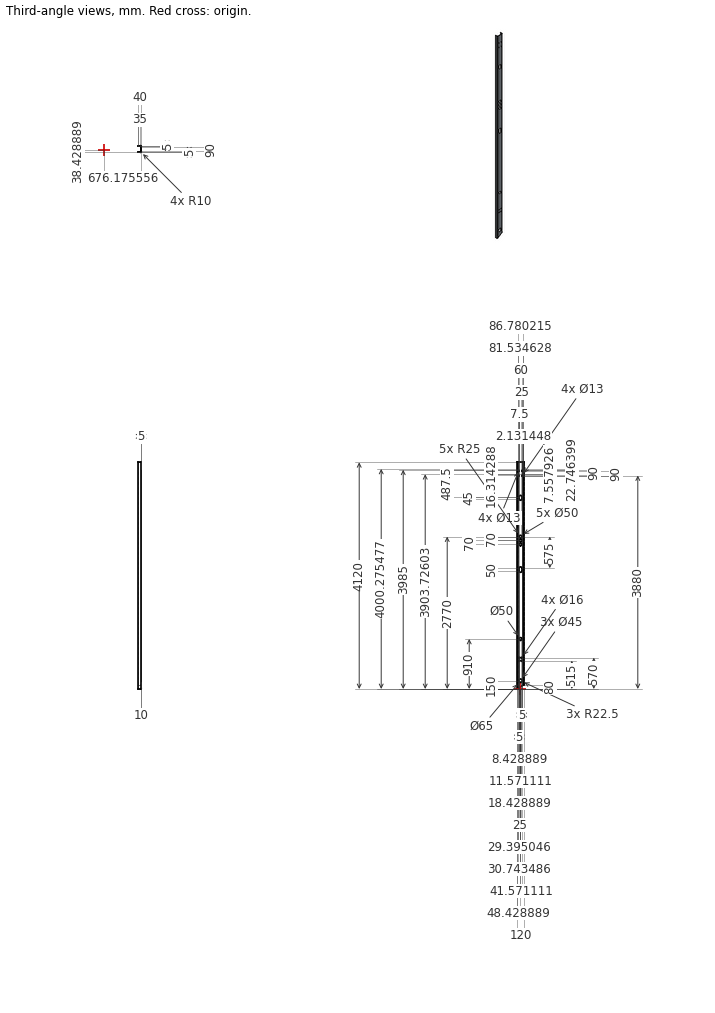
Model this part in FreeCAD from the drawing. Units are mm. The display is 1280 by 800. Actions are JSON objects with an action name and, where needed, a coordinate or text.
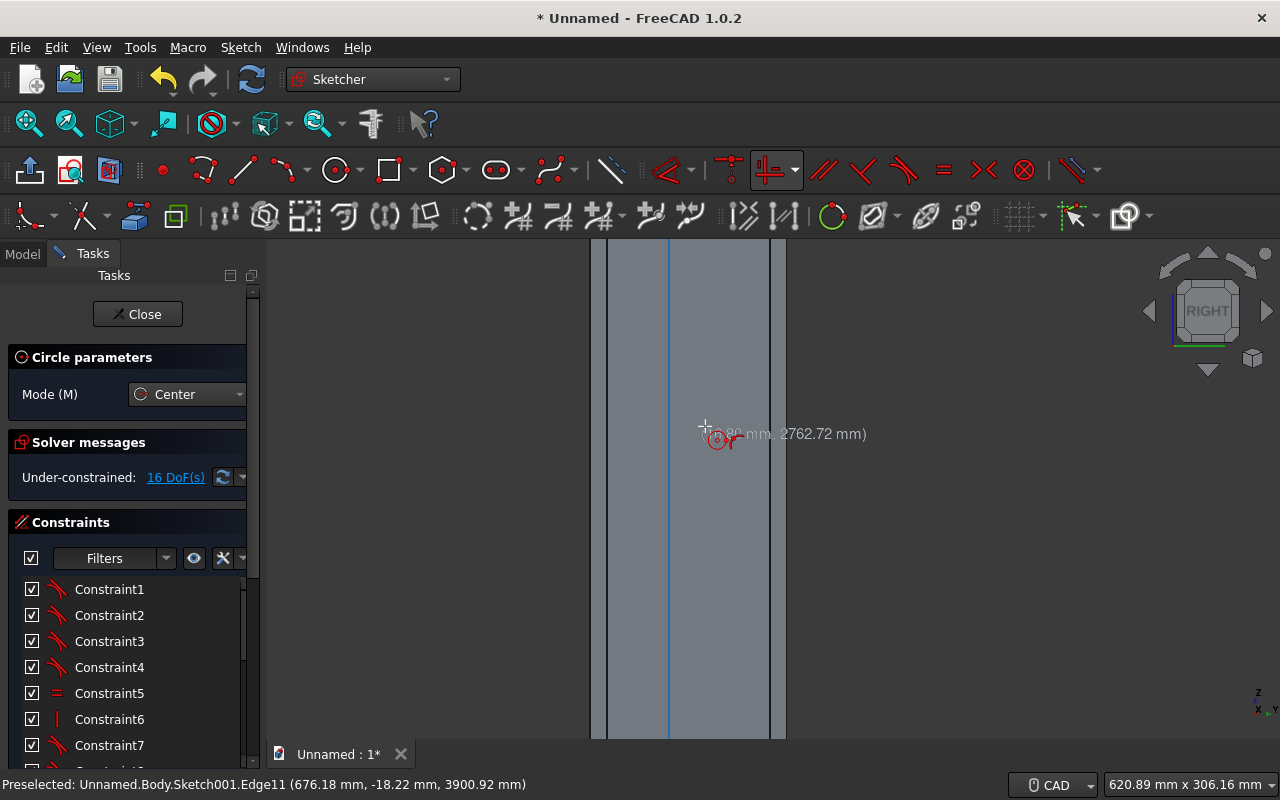
{"action": "left_click", "coordinate": [688, 427]}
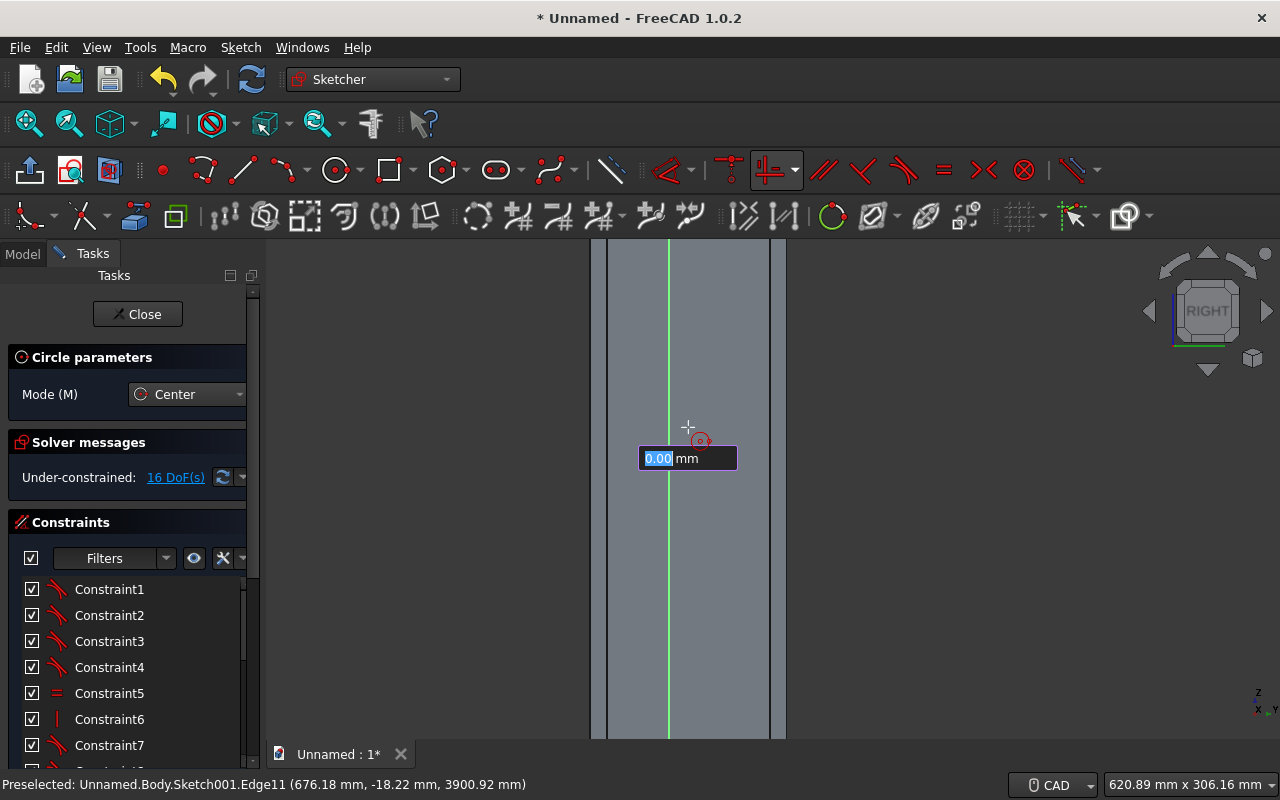
{"action": "scroll", "coordinate": [705, 426], "scroll_direction": "down", "scroll_amount": 15}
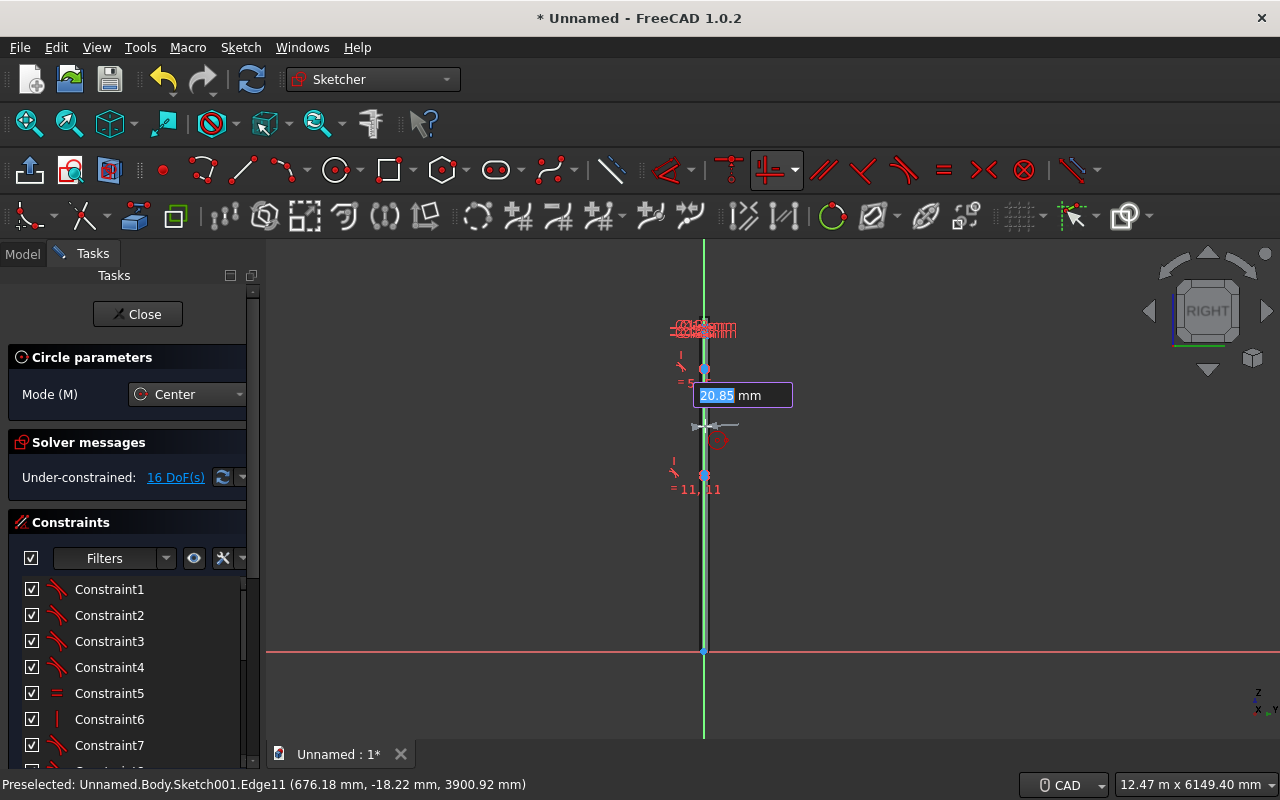
{"action": "scroll", "coordinate": [706, 425], "scroll_direction": "up", "scroll_amount": 10}
{"action": "mouse_move", "coordinate": [703, 422]}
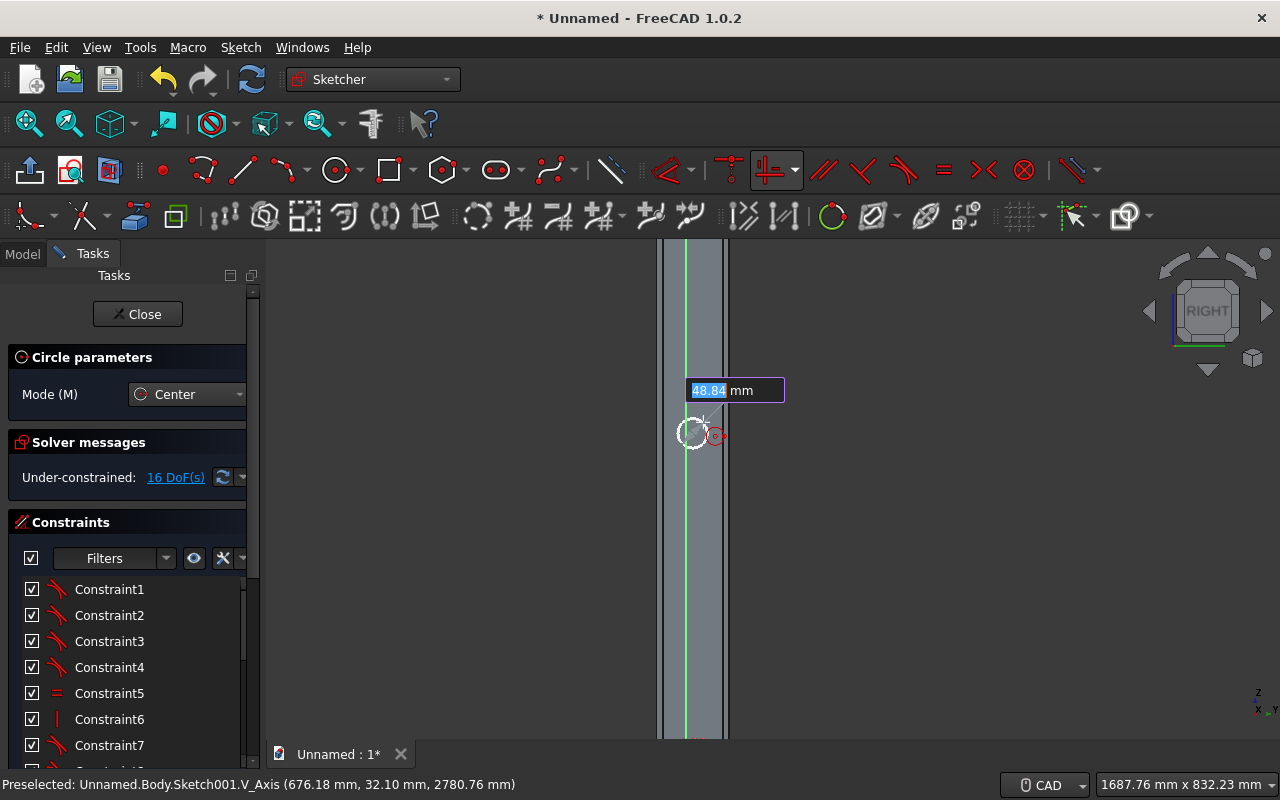
{"action": "type", "text": "50"}
{"action": "key", "text": "Return"}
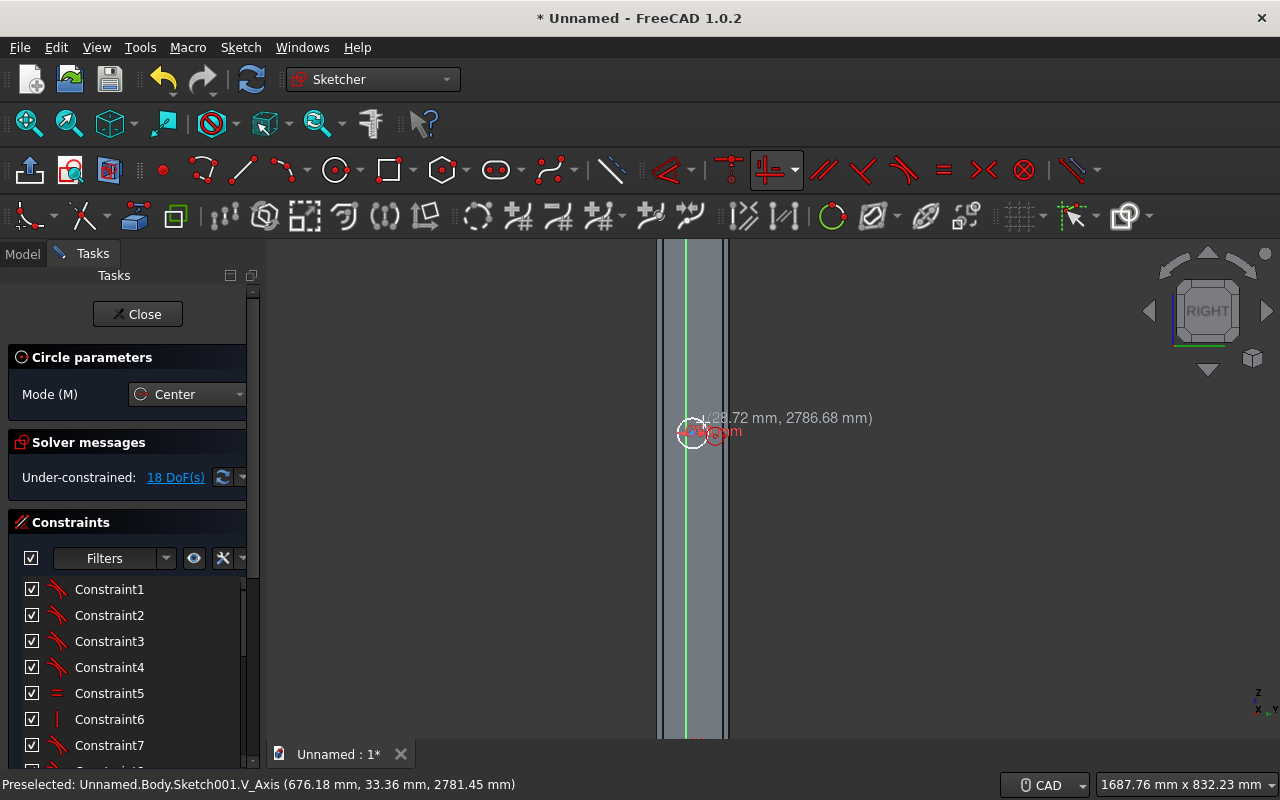
{"action": "scroll", "coordinate": [693, 475], "scroll_direction": "up", "scroll_amount": 5}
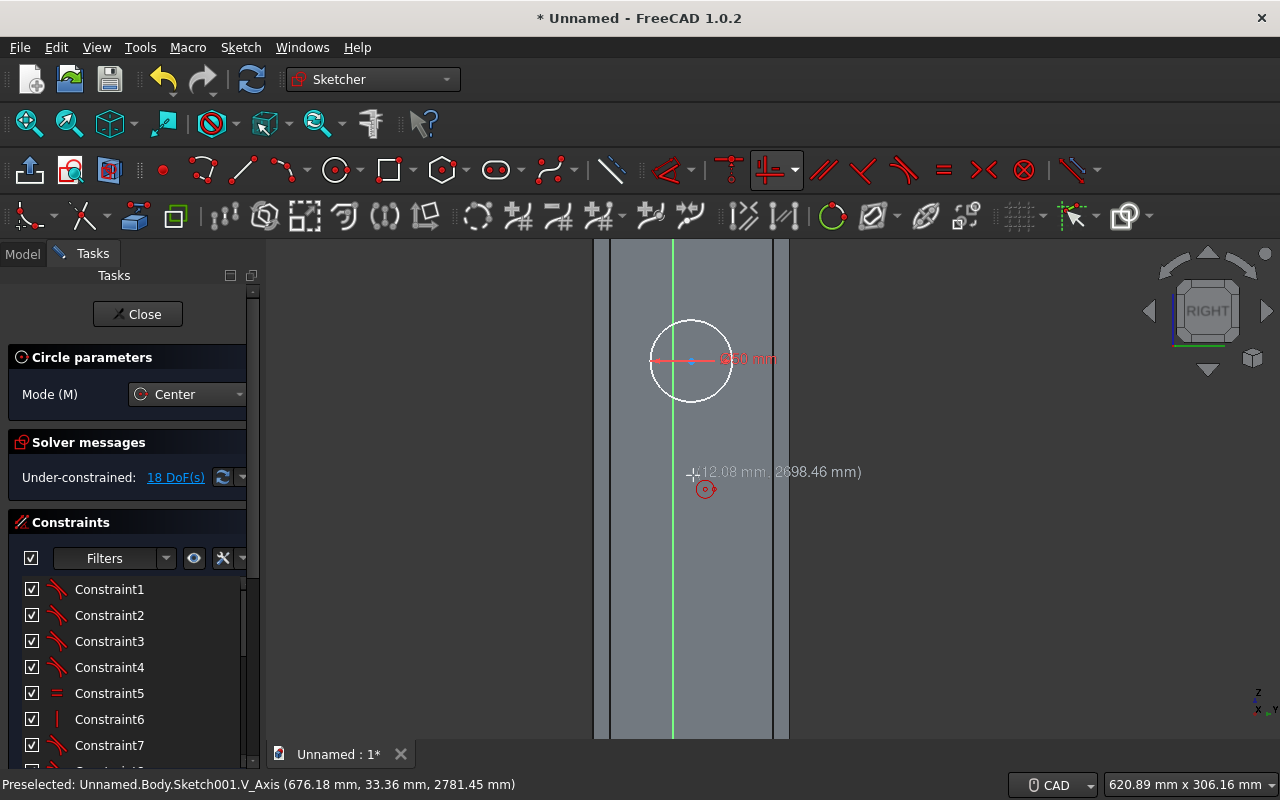
{"action": "left_click", "coordinate": [691, 474]}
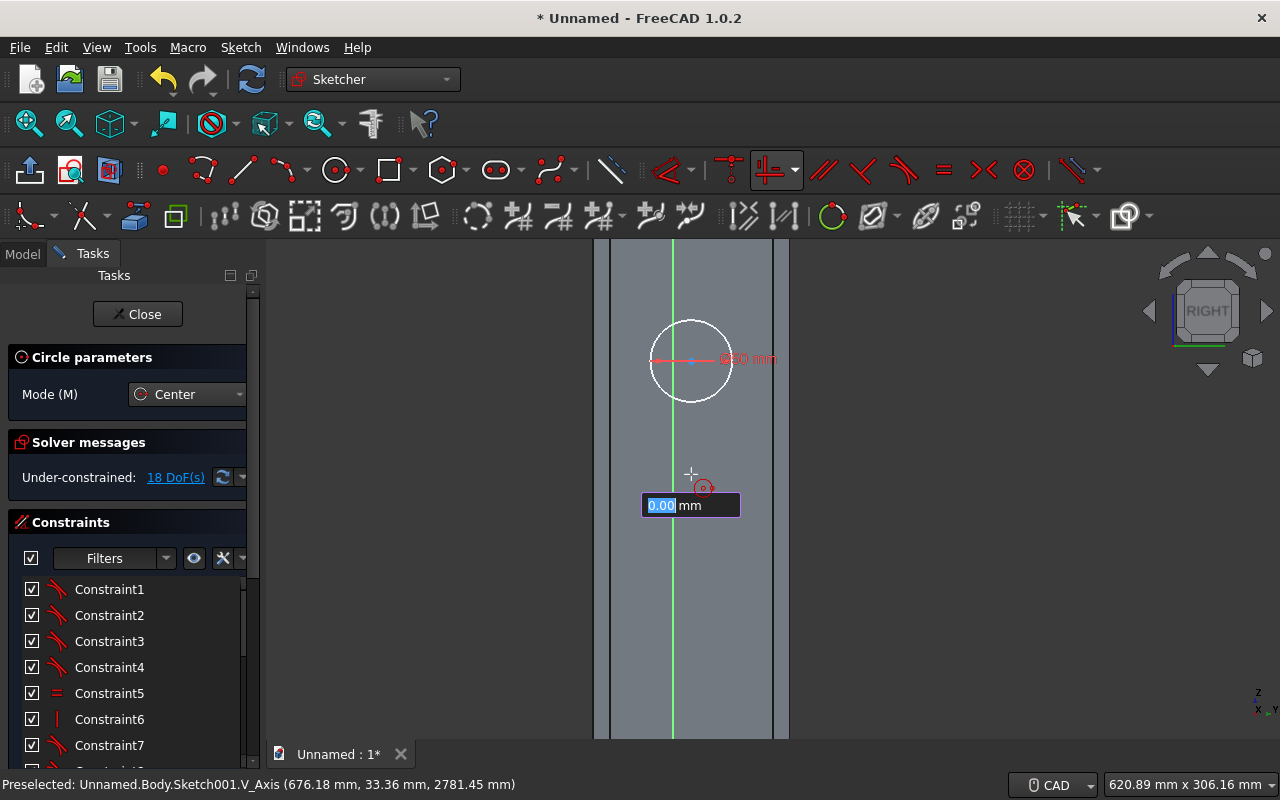
{"action": "scroll", "coordinate": [705, 430], "scroll_direction": "down", "scroll_amount": 15}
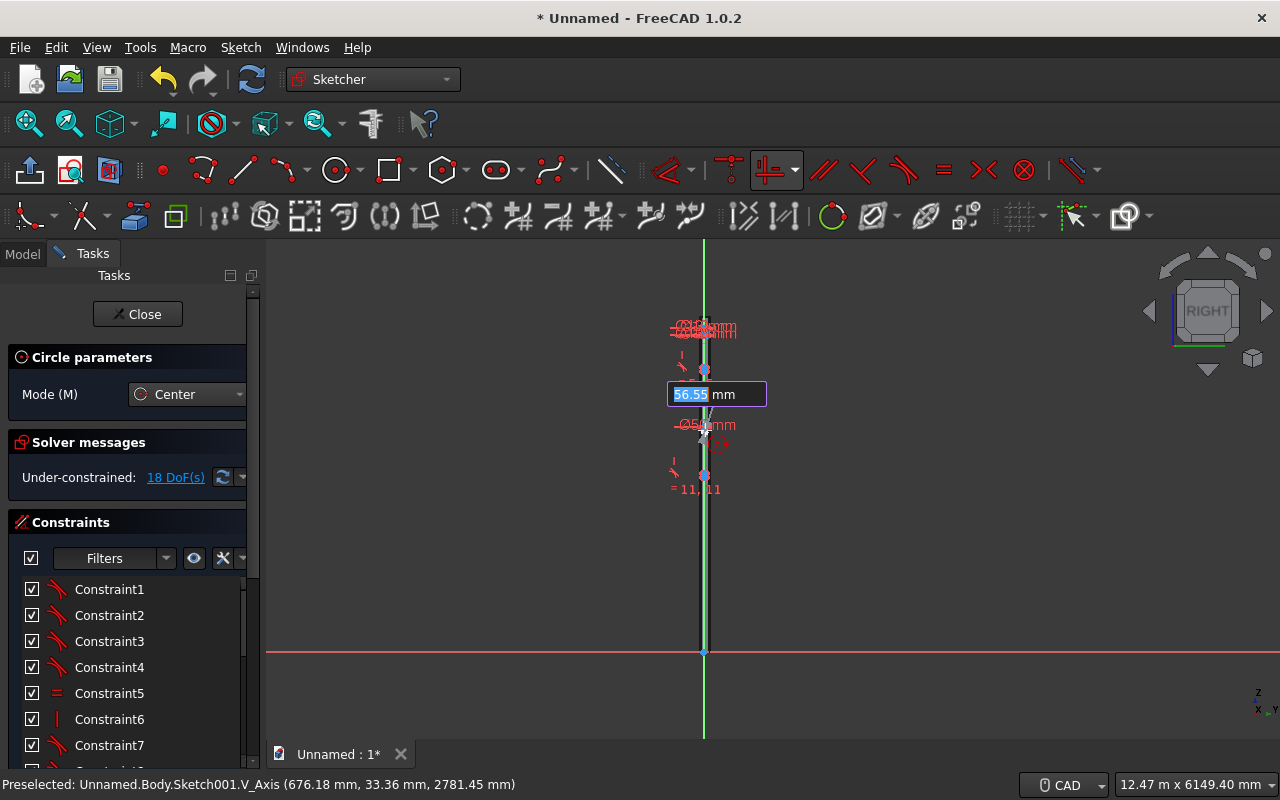
{"action": "scroll", "coordinate": [706, 431], "scroll_direction": "up", "scroll_amount": 10}
{"action": "mouse_move", "coordinate": [705, 430]}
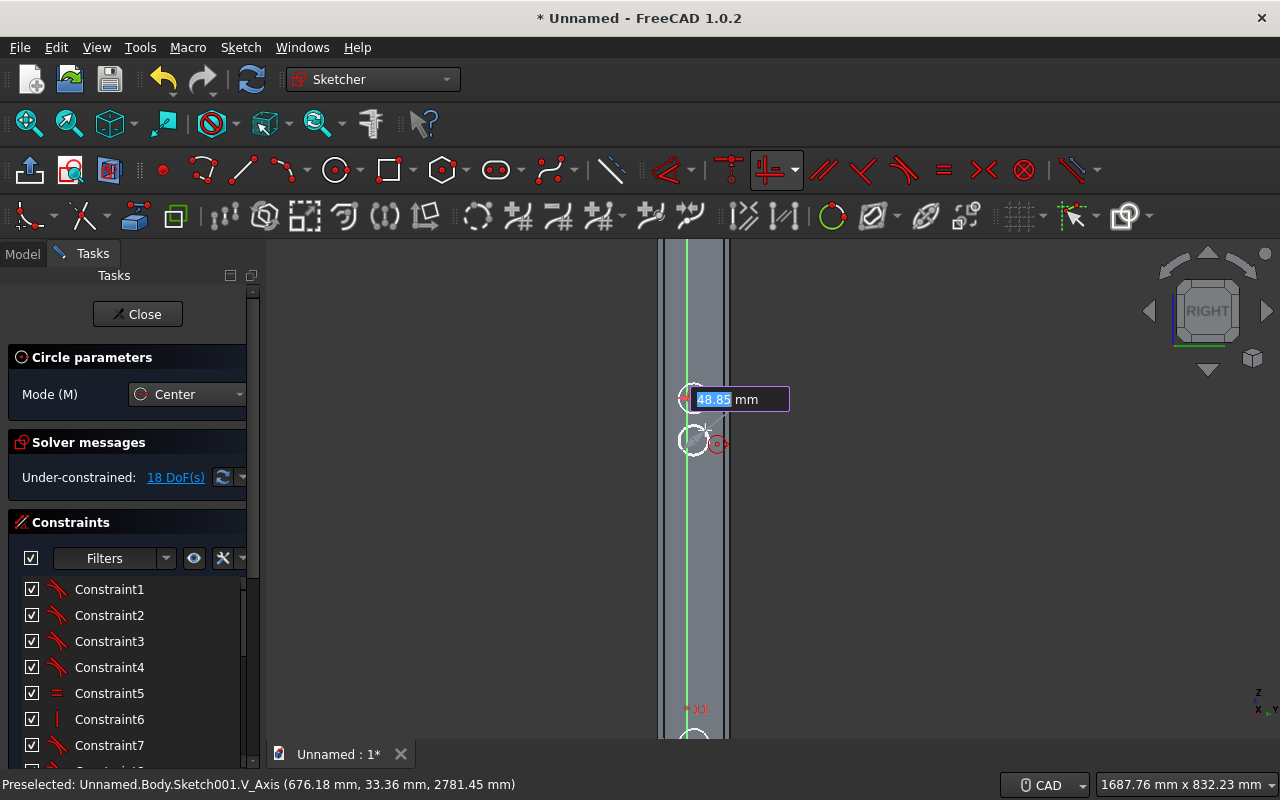
{"action": "type", "text": "50"}
{"action": "key", "text": "Return"}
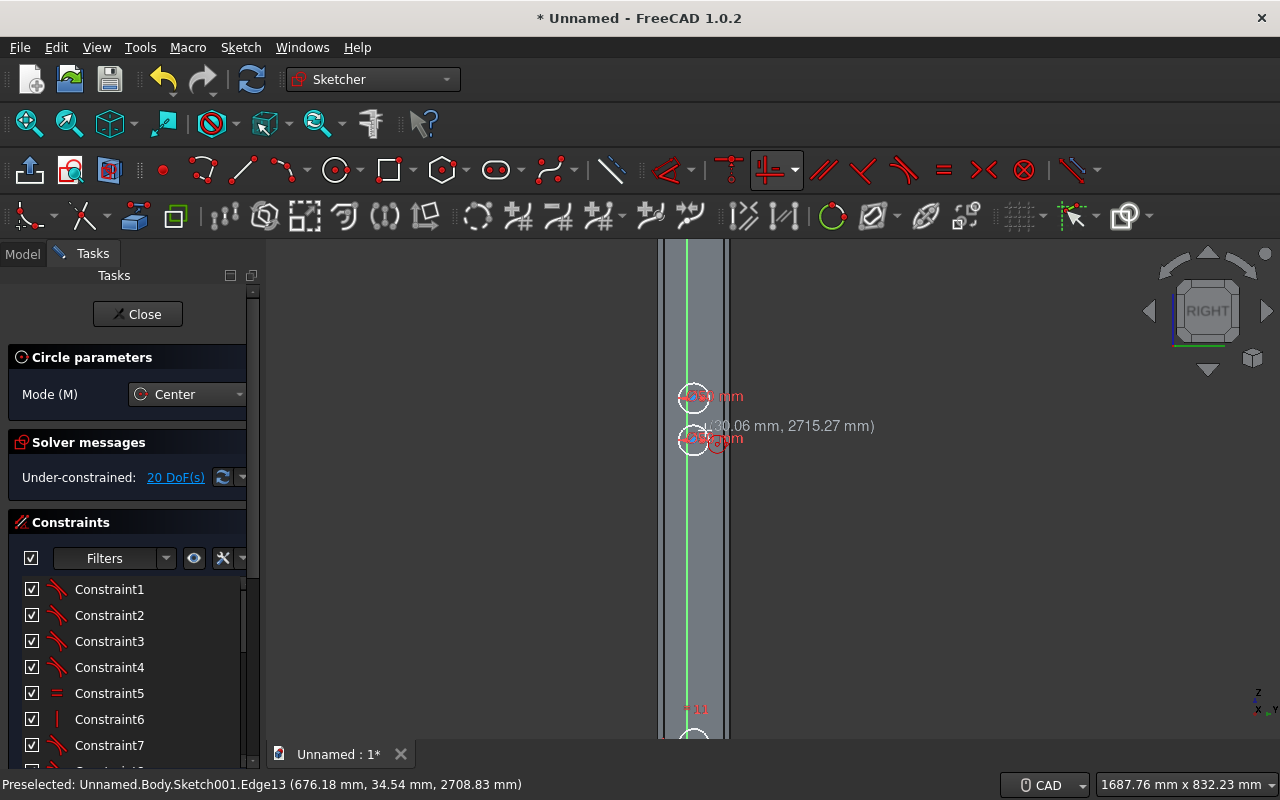
{"action": "scroll", "coordinate": [694, 482], "scroll_direction": "up", "scroll_amount": 5}